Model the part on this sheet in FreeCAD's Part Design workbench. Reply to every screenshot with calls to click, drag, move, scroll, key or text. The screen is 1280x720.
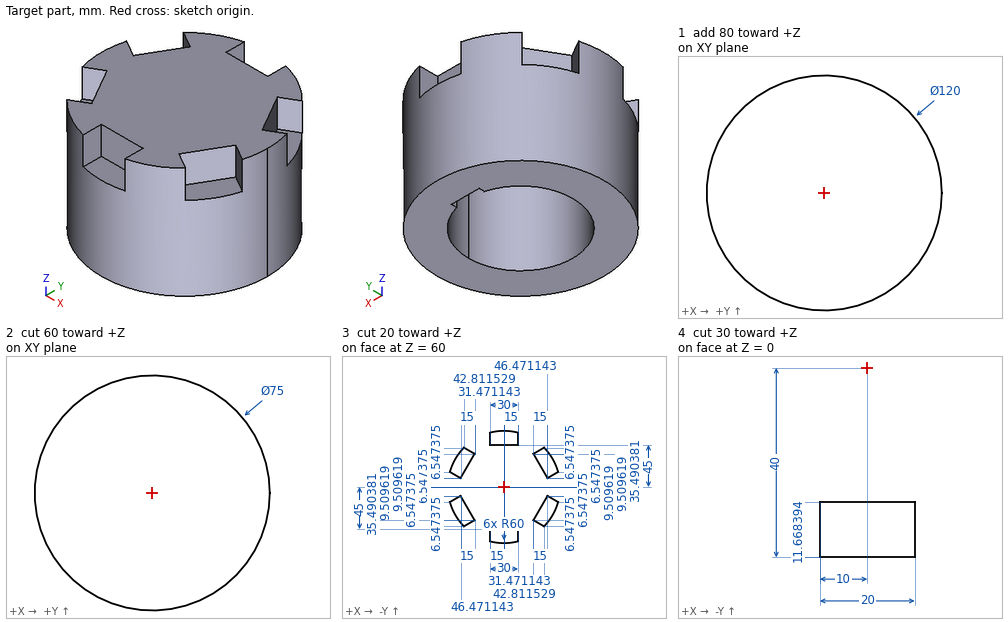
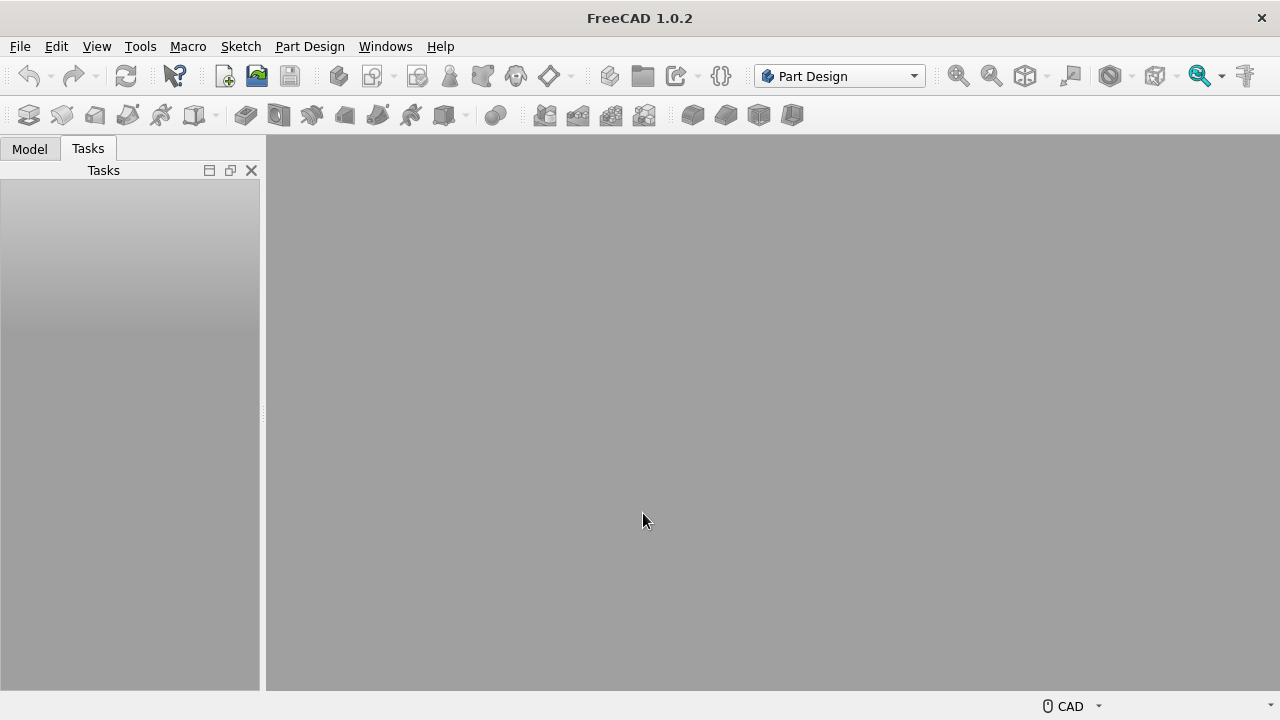
click(224, 76)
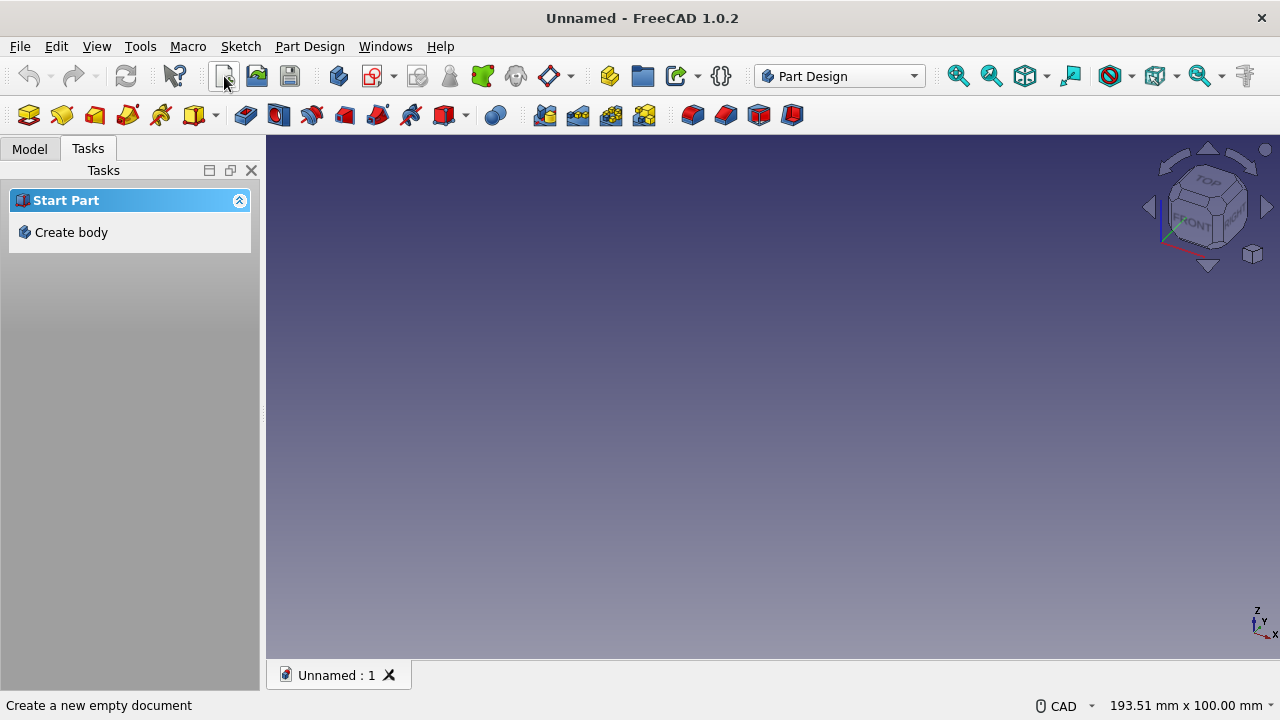
click(372, 76)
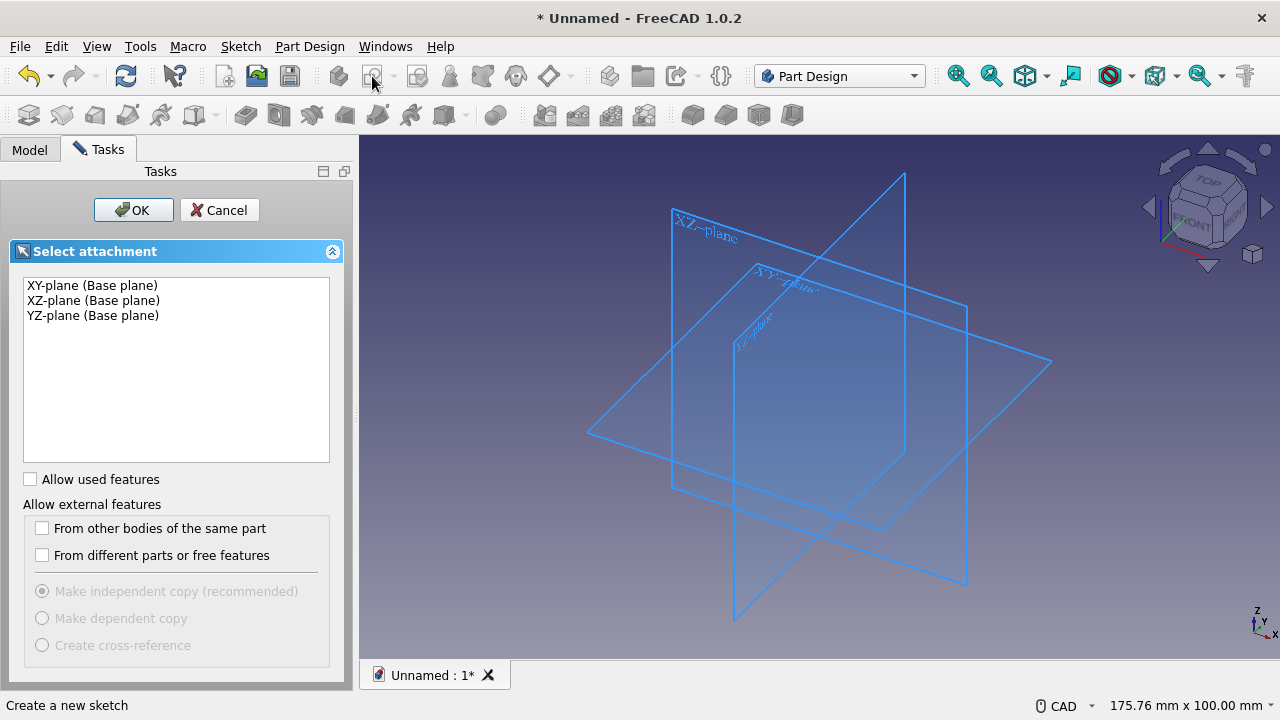
click(84, 286)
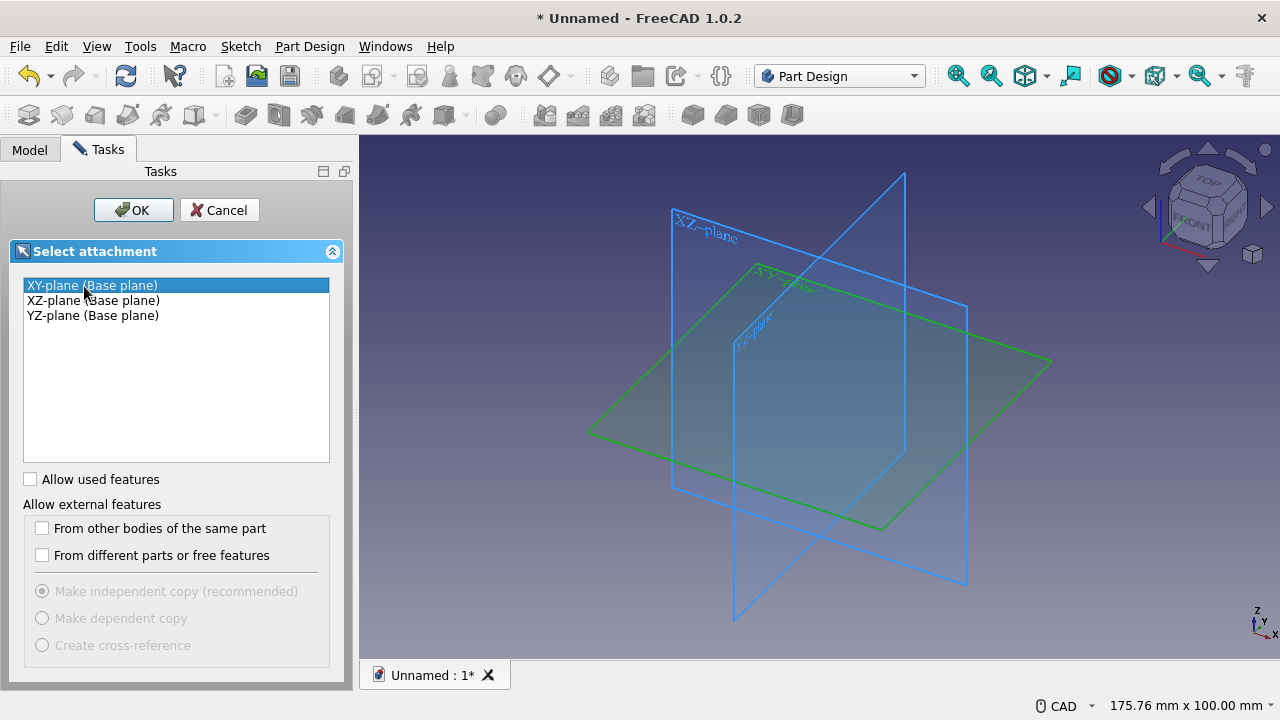
click(134, 210)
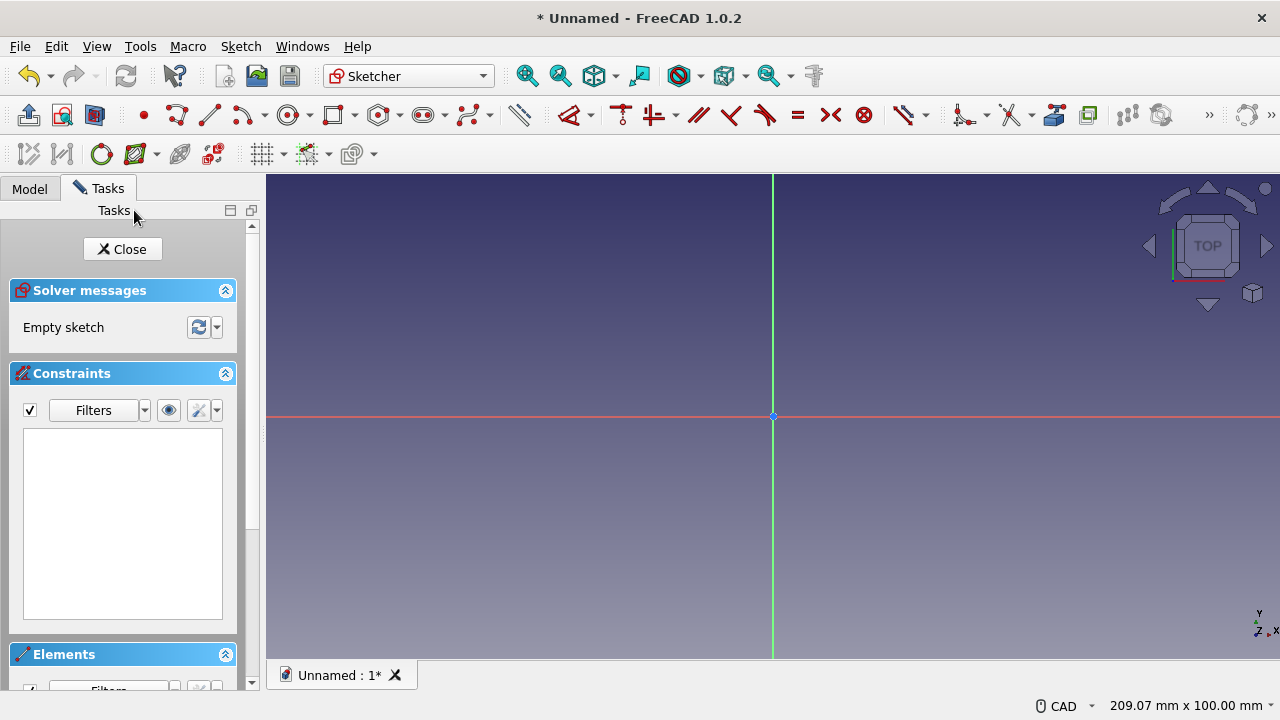
scroll(621, 416, down, 3)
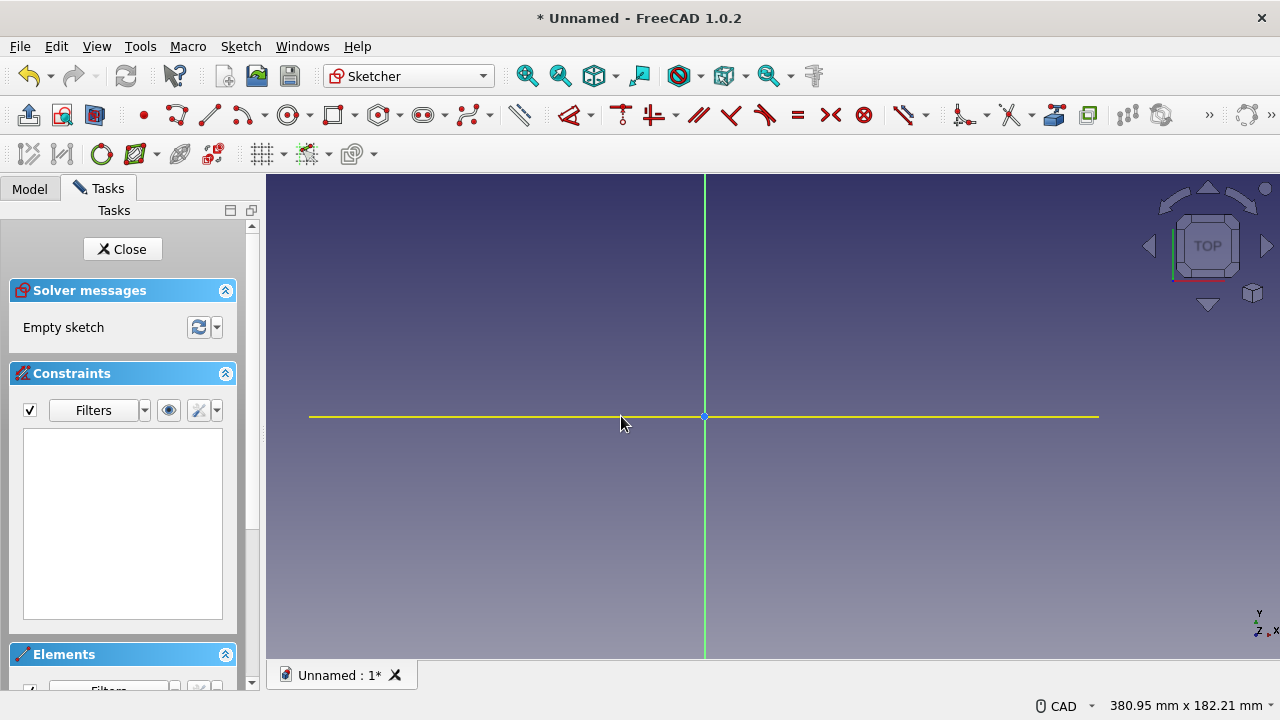
click(288, 116)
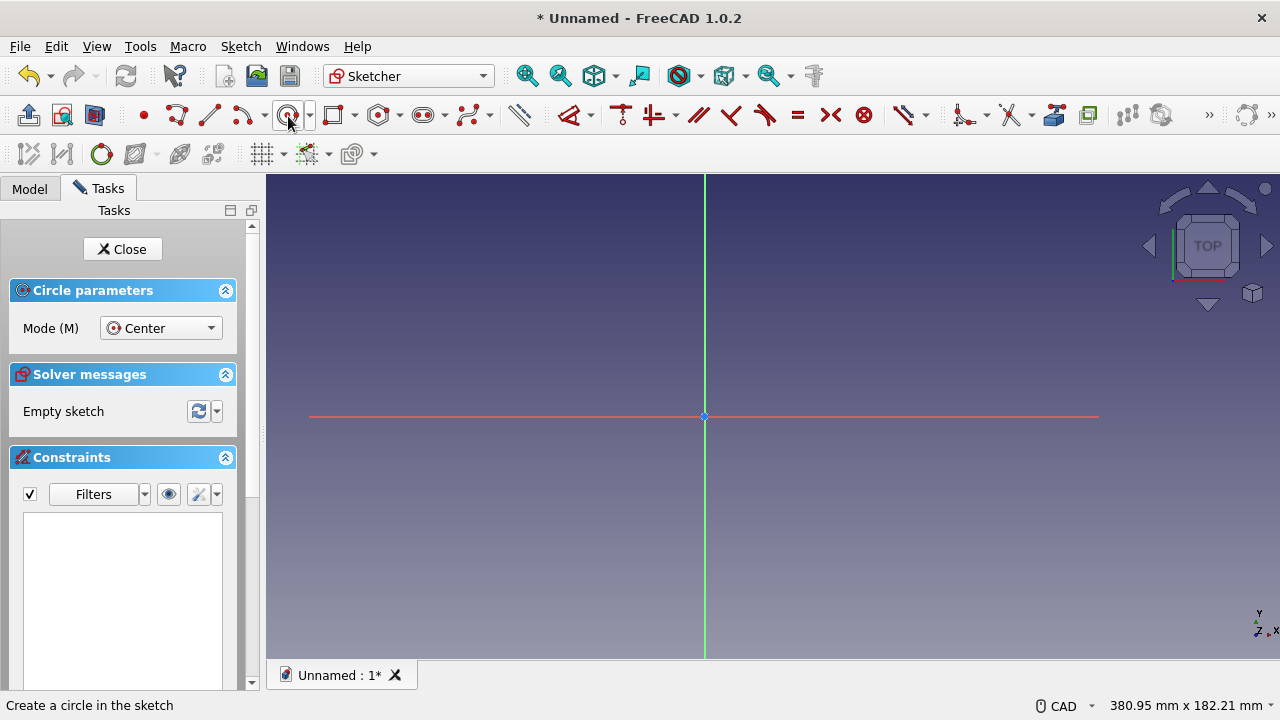
click(705, 416)
click(818, 304)
key(Escape)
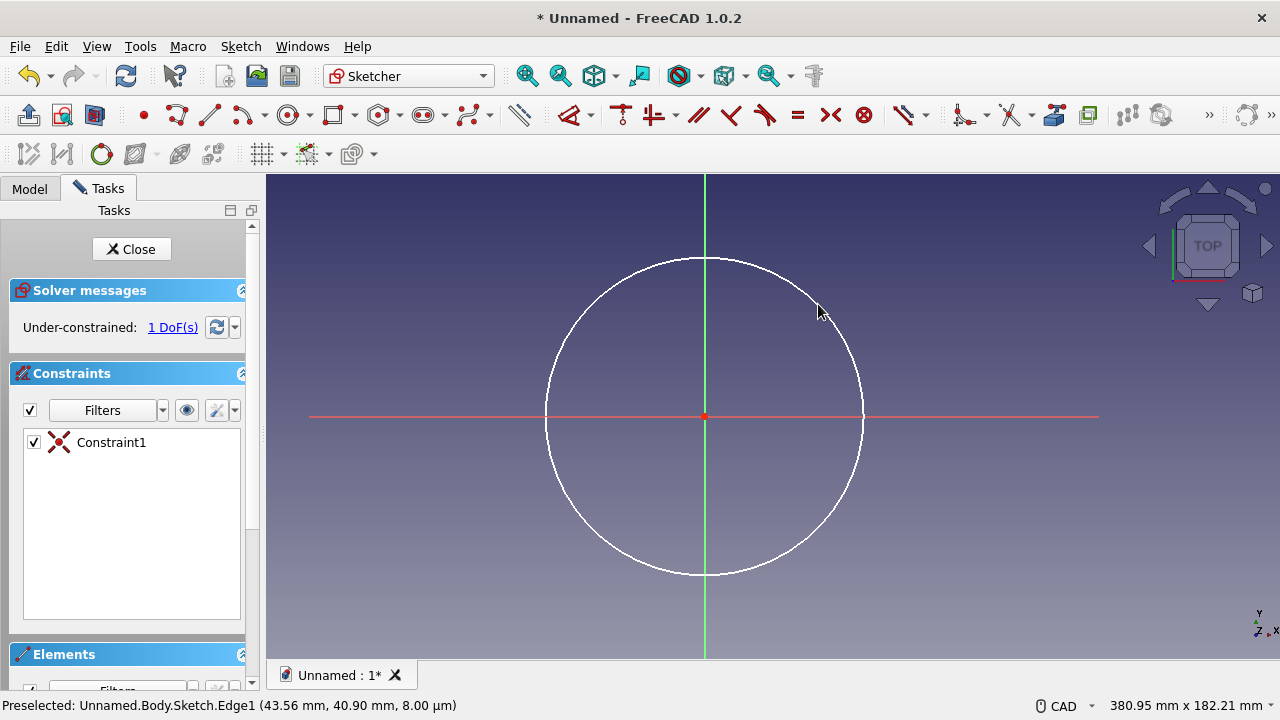
click(568, 116)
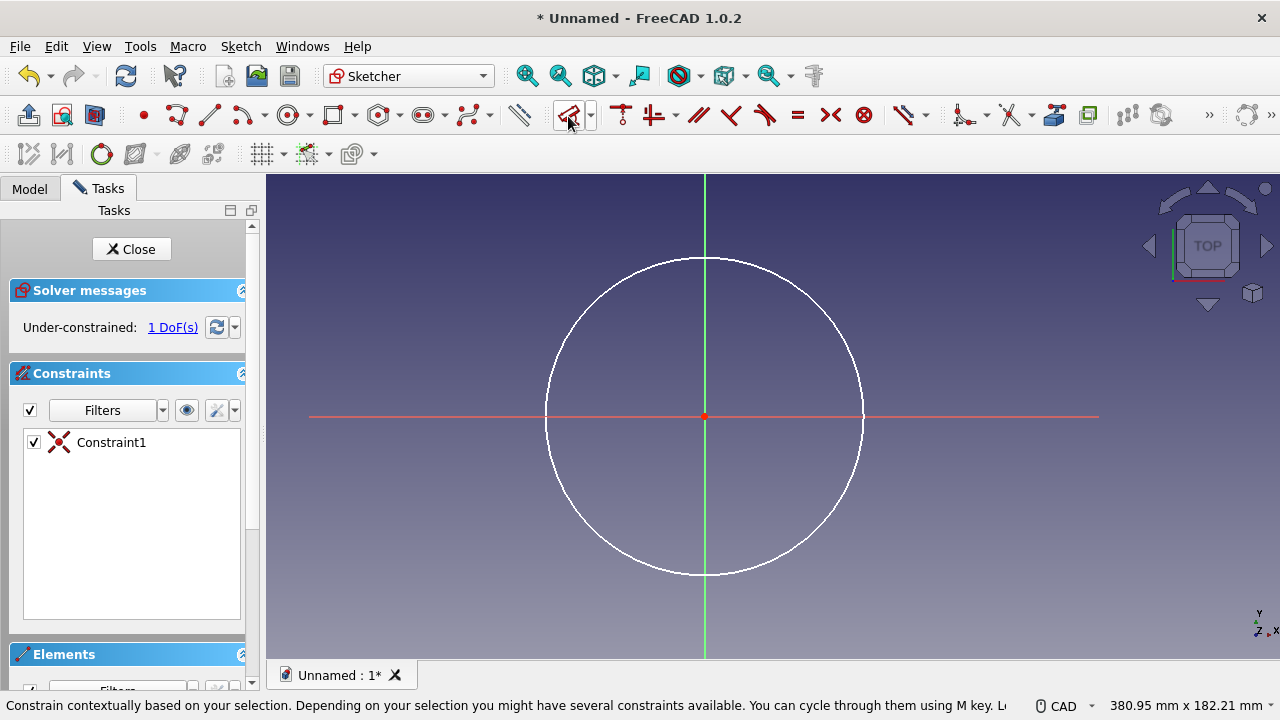
click(817, 304)
click(840, 281)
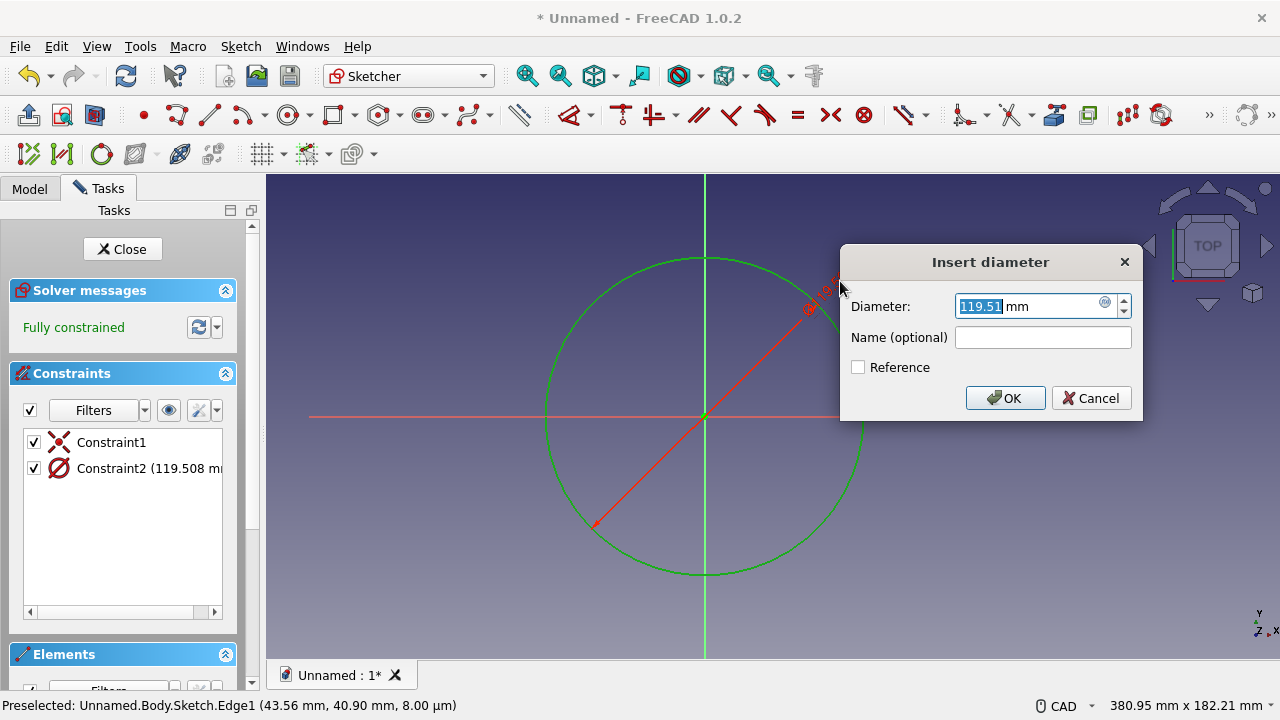
text(120)
key(Return)
key(Escape)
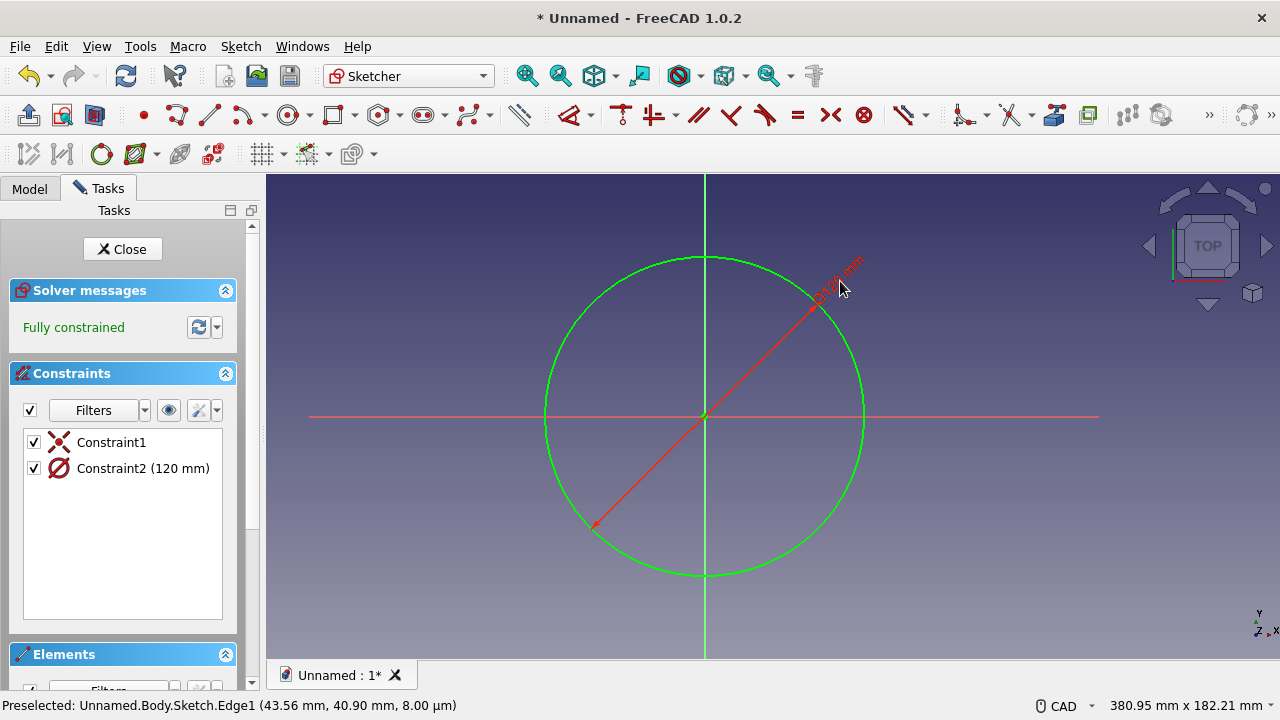
click(123, 249)